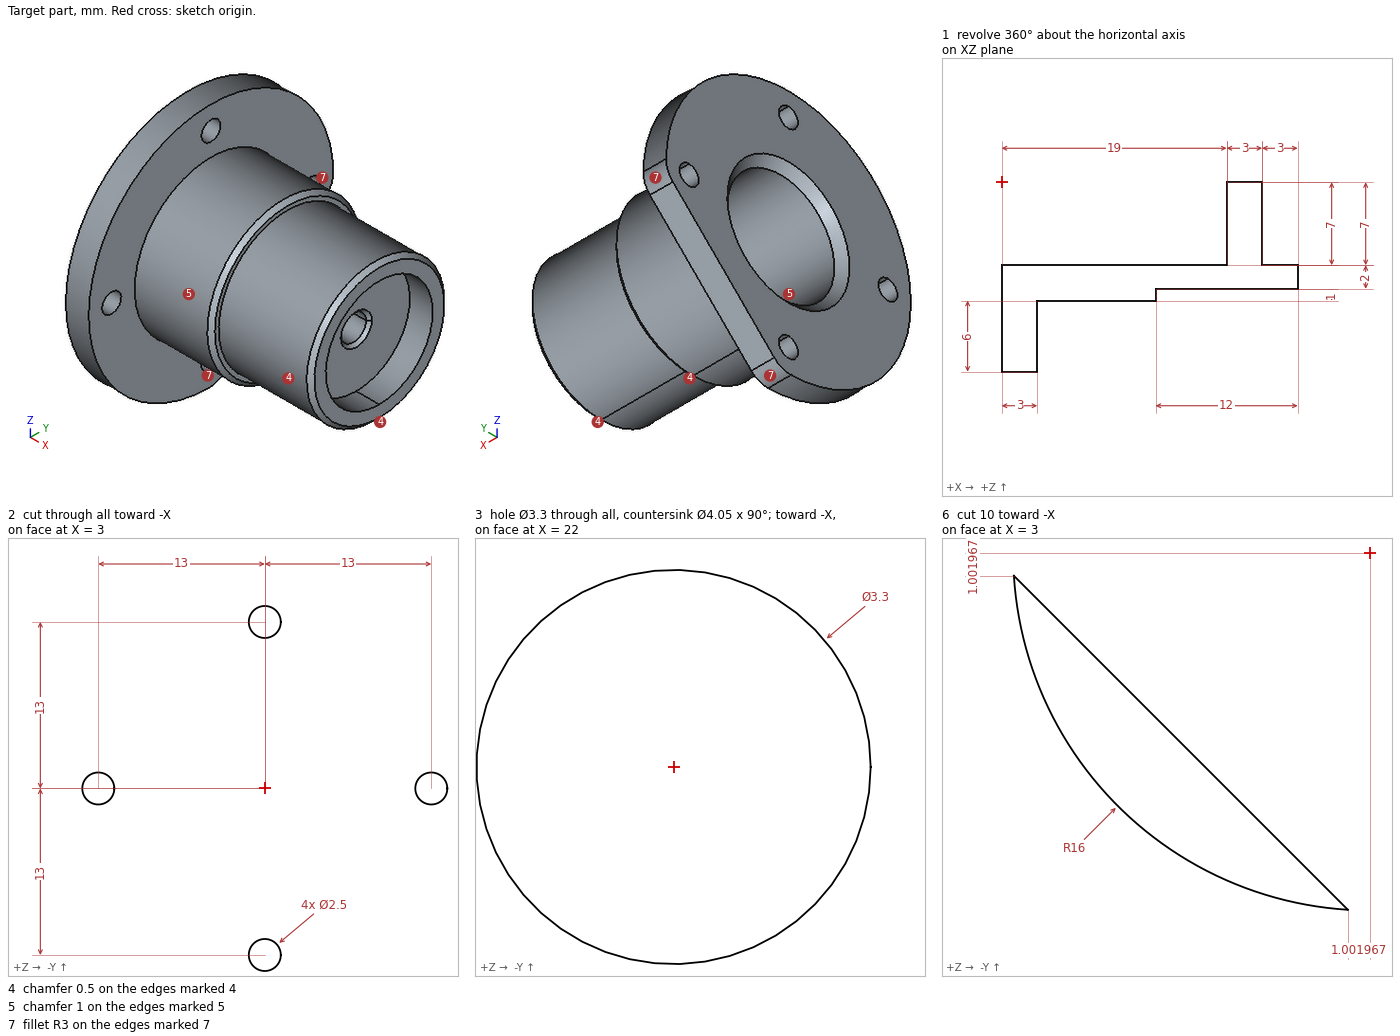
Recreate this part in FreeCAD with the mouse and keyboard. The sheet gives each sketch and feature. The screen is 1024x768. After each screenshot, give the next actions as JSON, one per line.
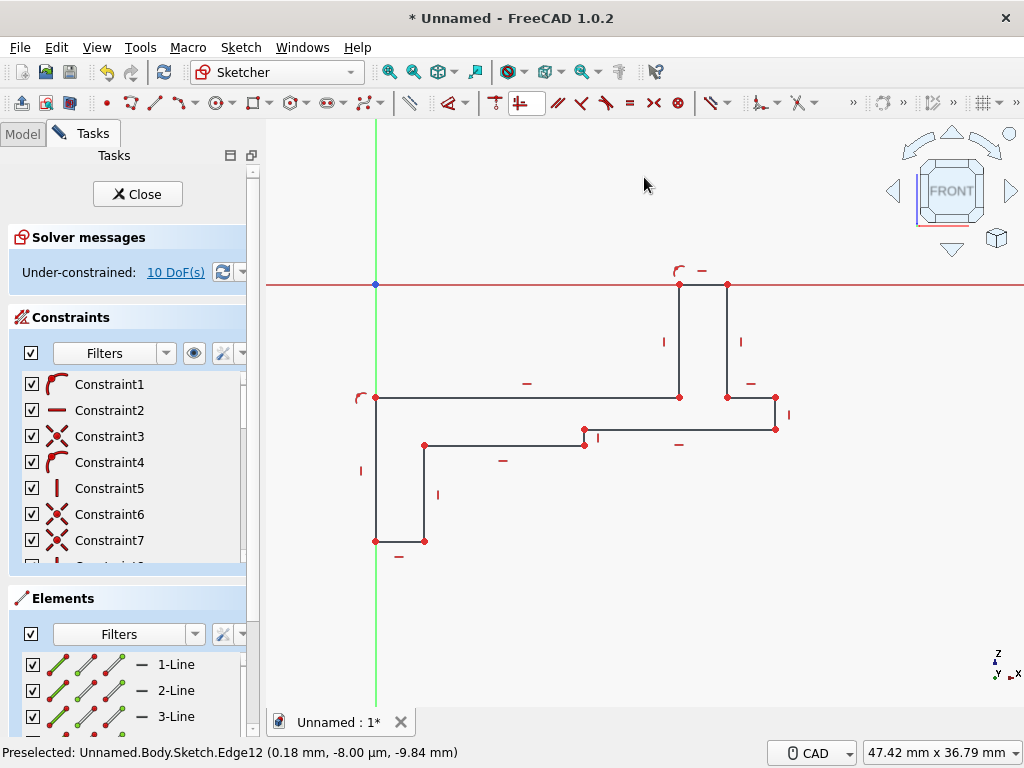
{"action": "left_click", "coordinate": [448, 104]}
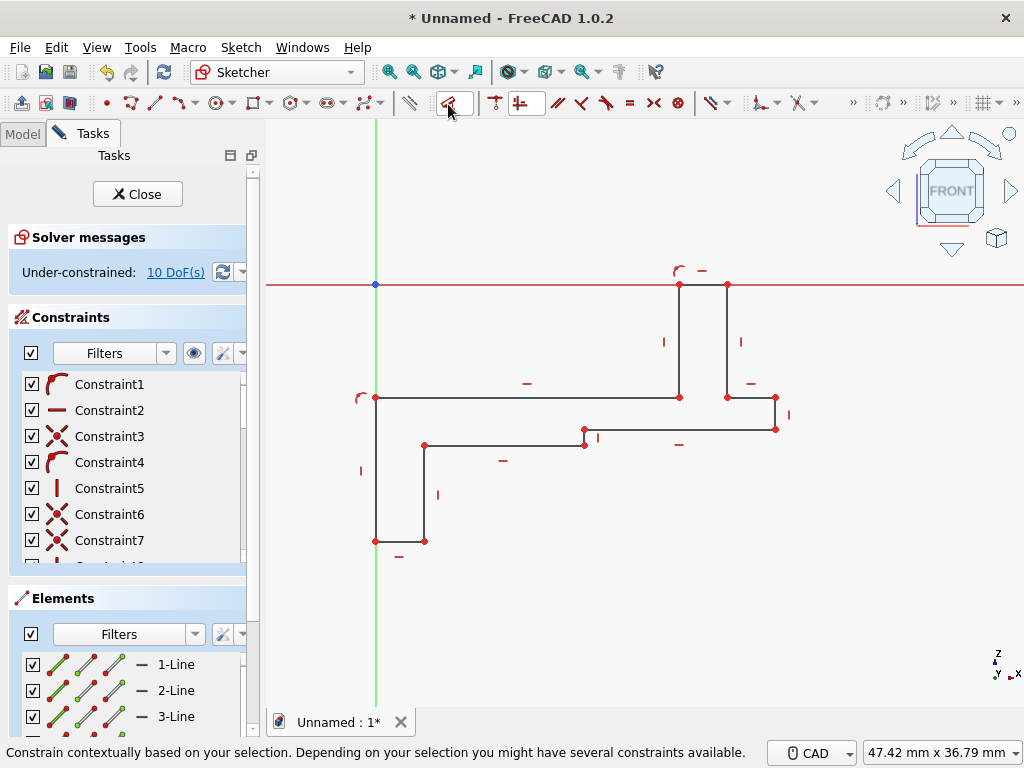
{"action": "left_click", "coordinate": [679, 364]}
{"action": "left_click", "coordinate": [713, 341]}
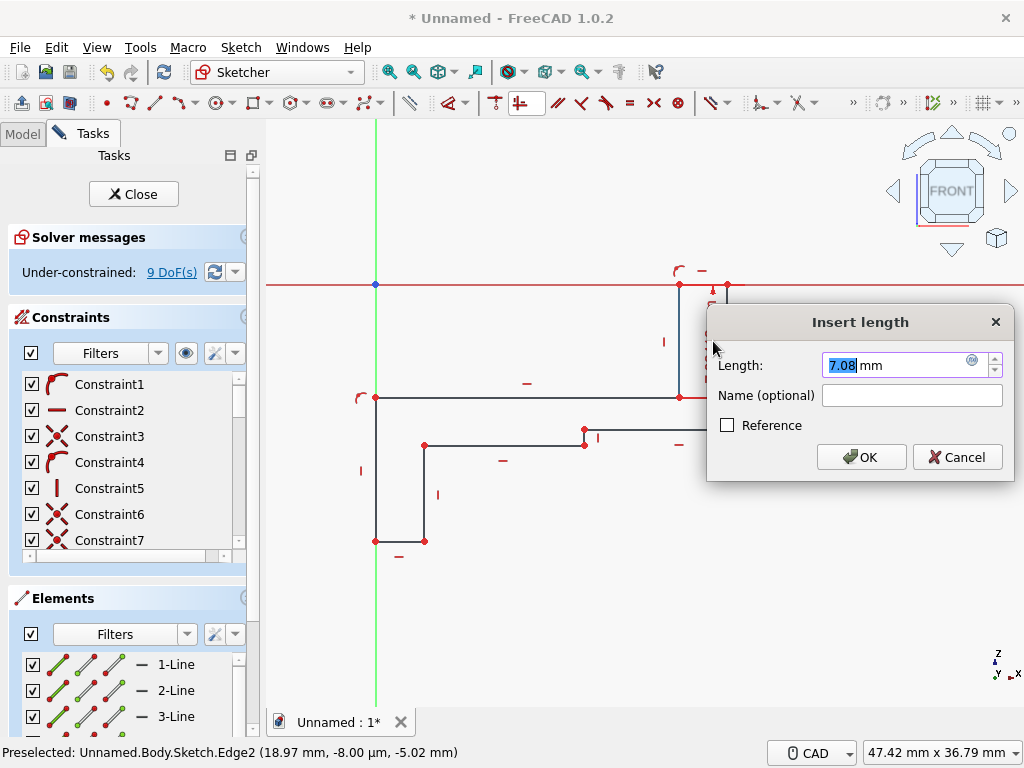
{"action": "type", "text": "7"}
{"action": "key", "text": "Return"}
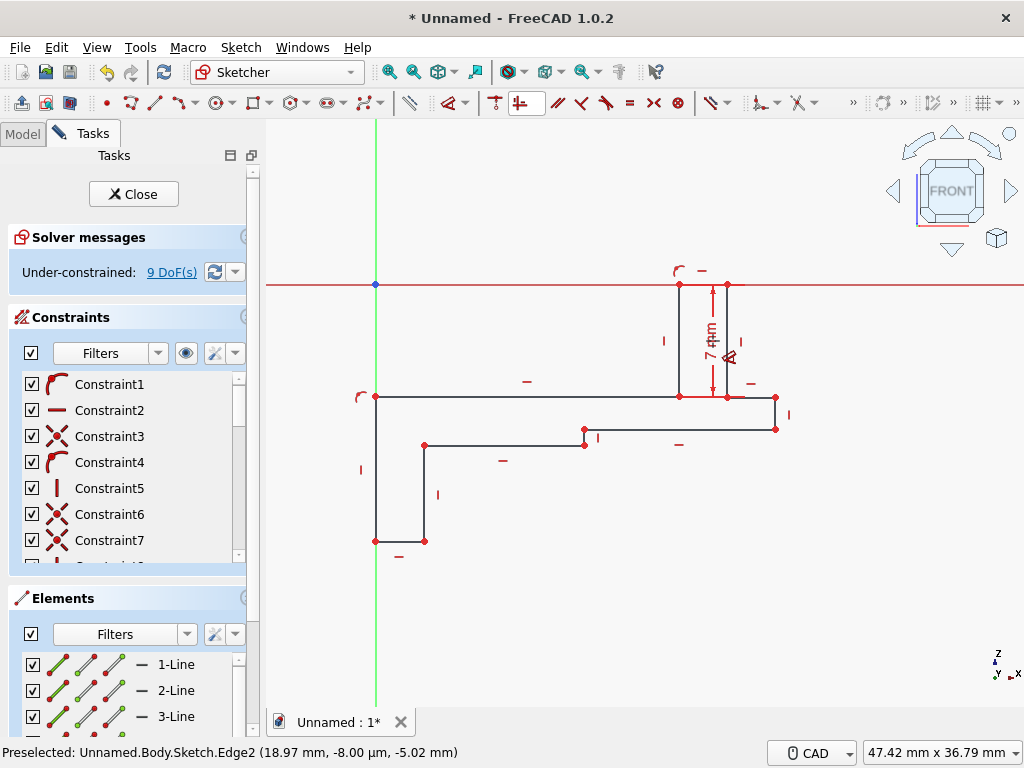
{"action": "left_click", "coordinate": [693, 285]}
{"action": "left_click", "coordinate": [703, 251]}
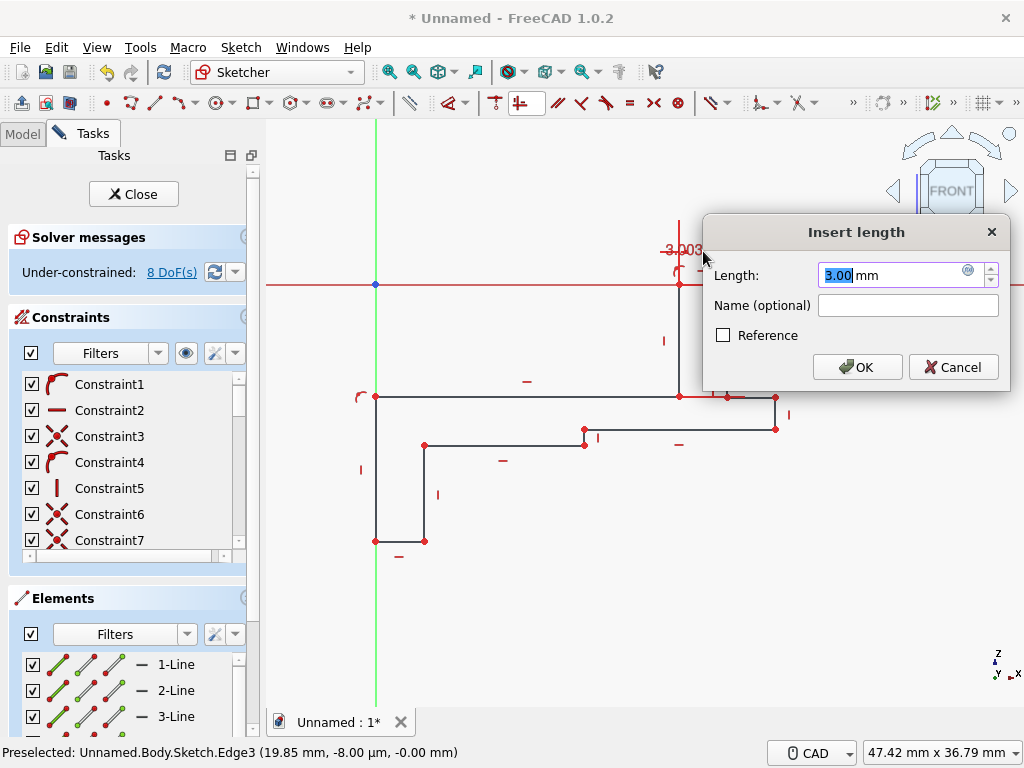
{"action": "type", "text": "3"}
{"action": "key", "text": "Return"}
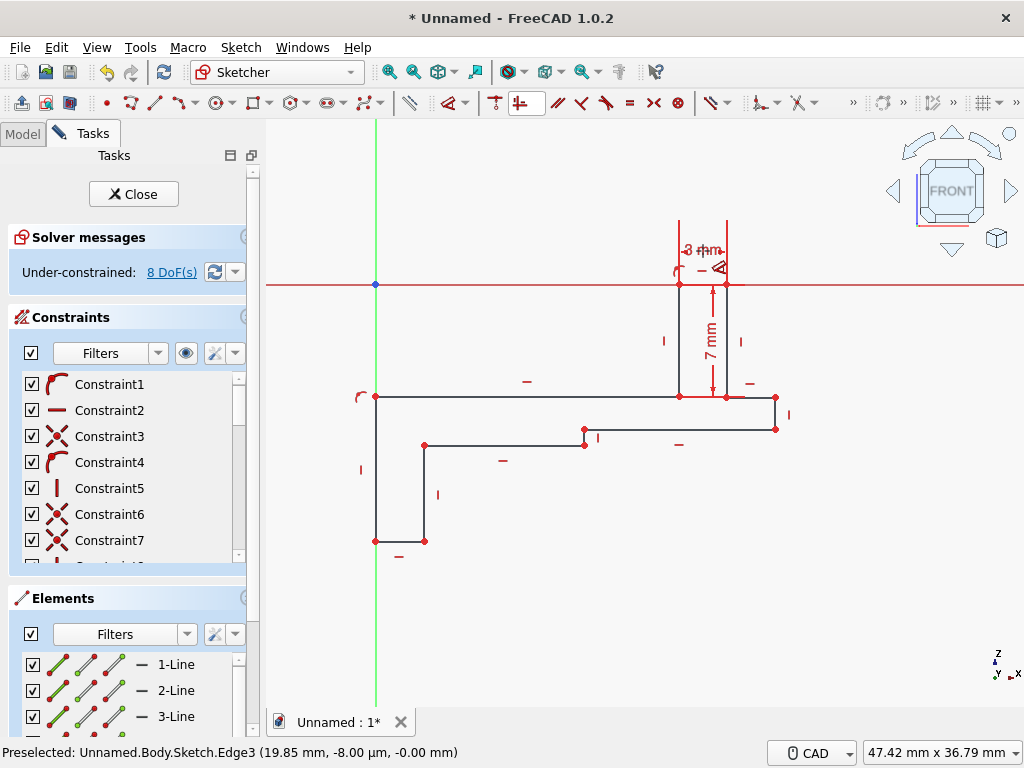
{"action": "left_click", "coordinate": [727, 319]}
{"action": "left_click", "coordinate": [761, 315]}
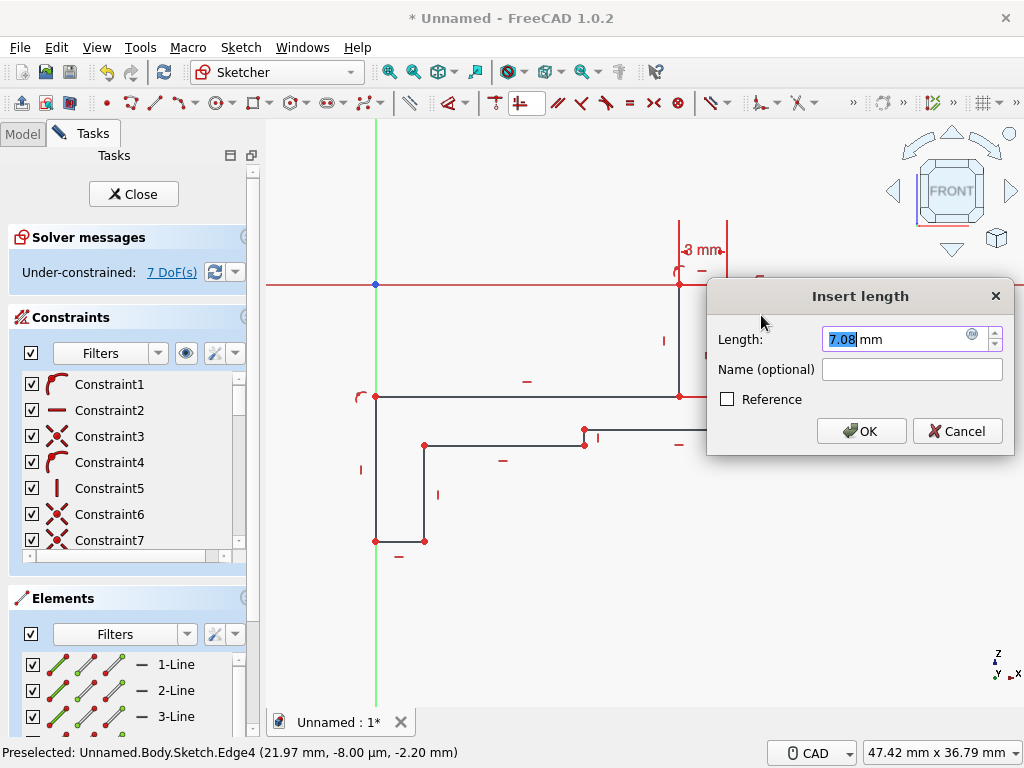
{"action": "type", "text": "7"}
{"action": "key", "text": "Return"}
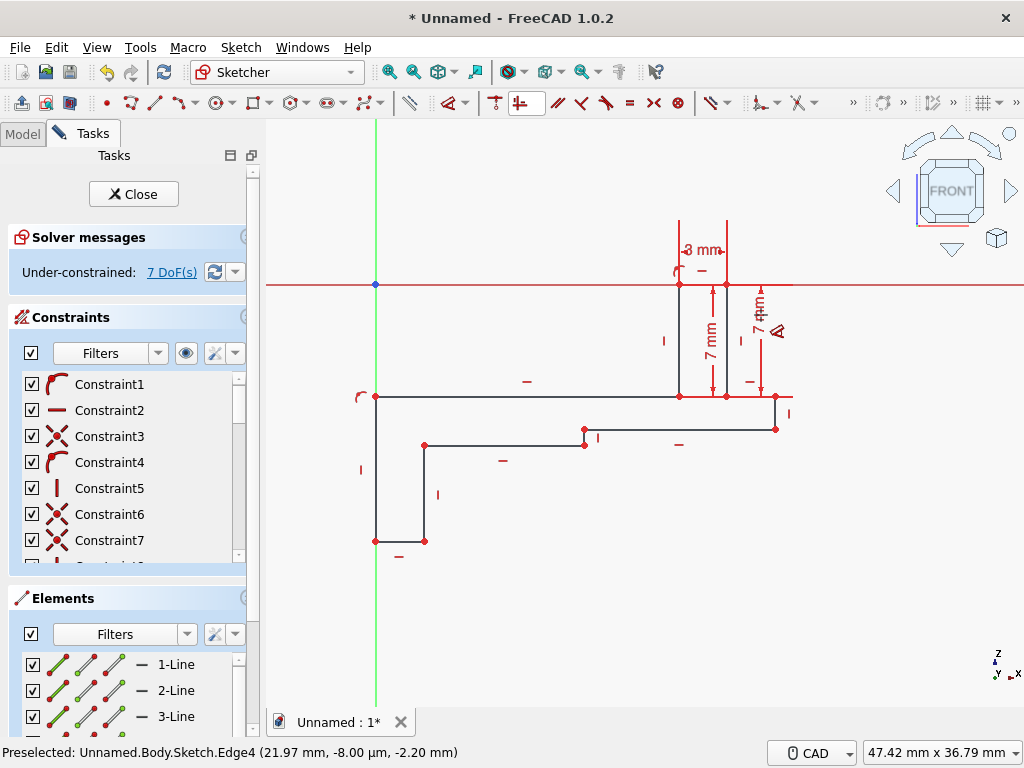
{"action": "left_click", "coordinate": [741, 397]}
{"action": "left_click", "coordinate": [751, 363]}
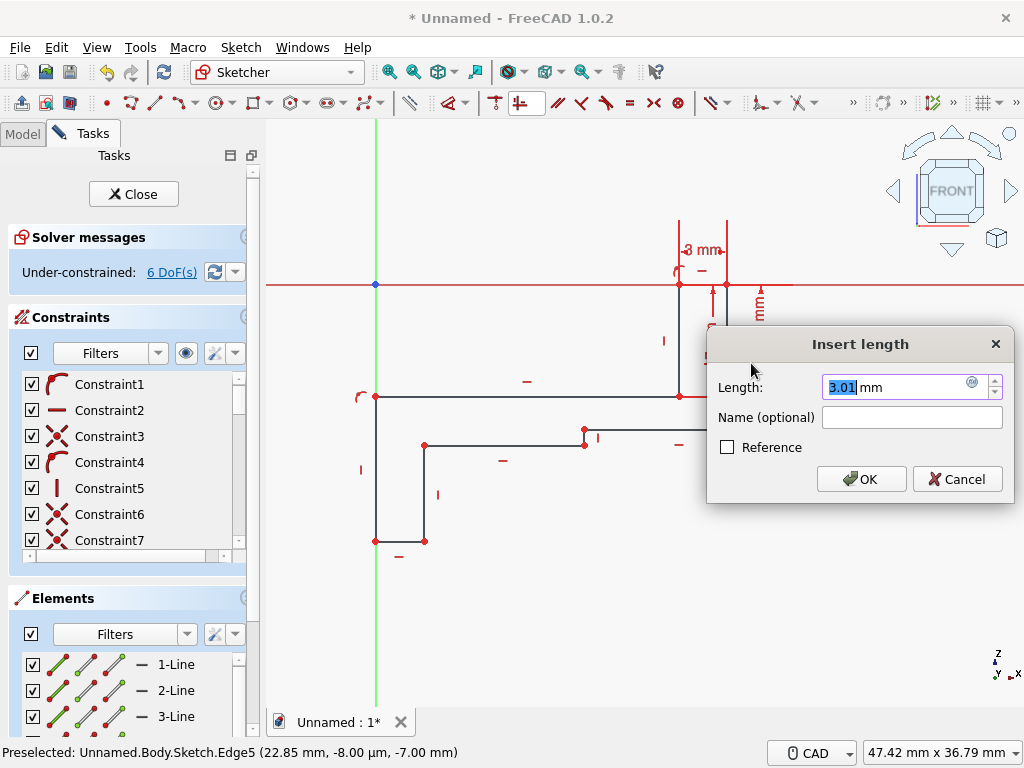
{"action": "type", "text": "3"}
{"action": "key", "text": "Return"}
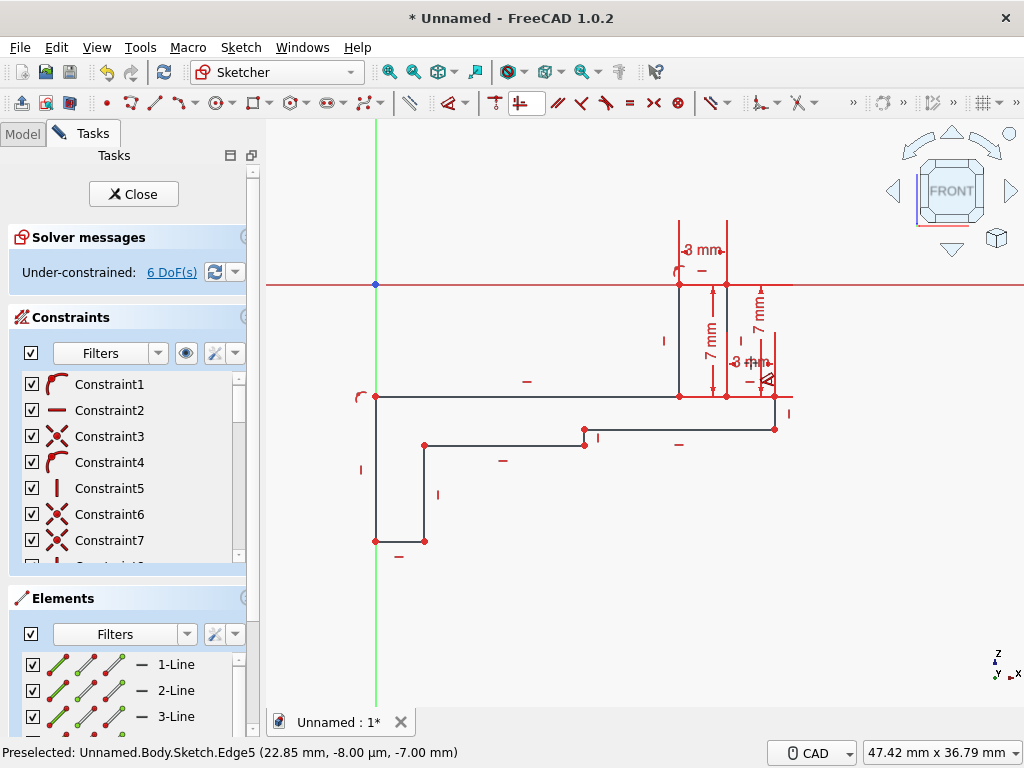
{"action": "scroll", "coordinate": [775, 407], "scroll_direction": "up", "scroll_amount": 2}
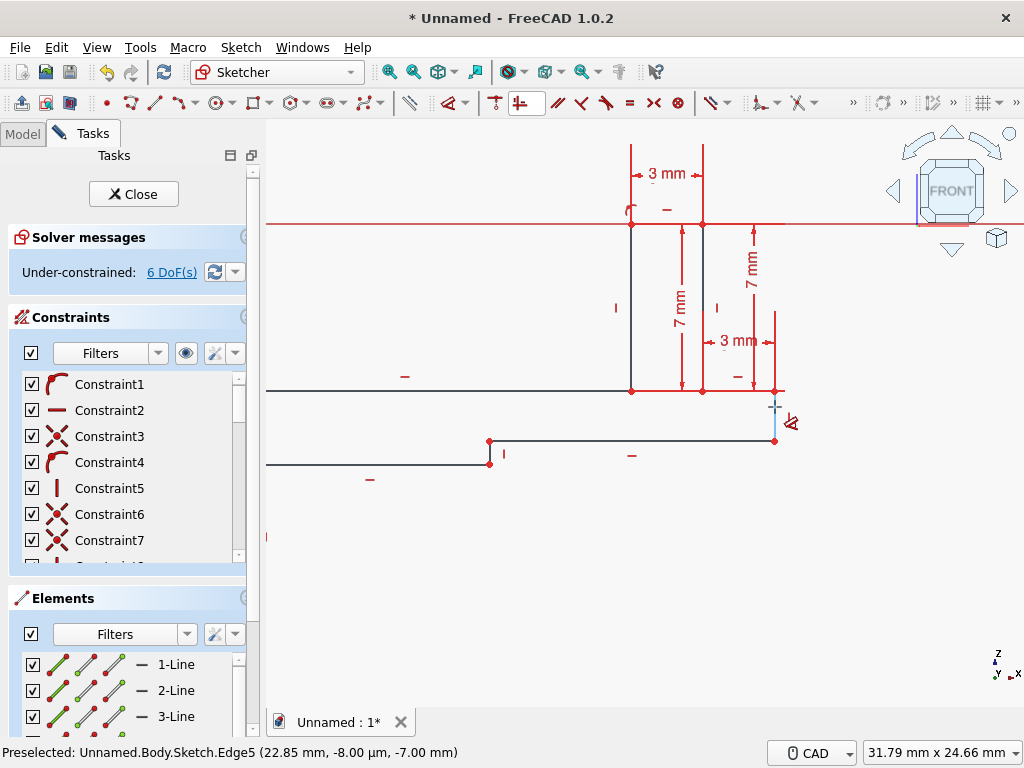
{"action": "left_click", "coordinate": [775, 406]}
{"action": "left_click", "coordinate": [809, 416]}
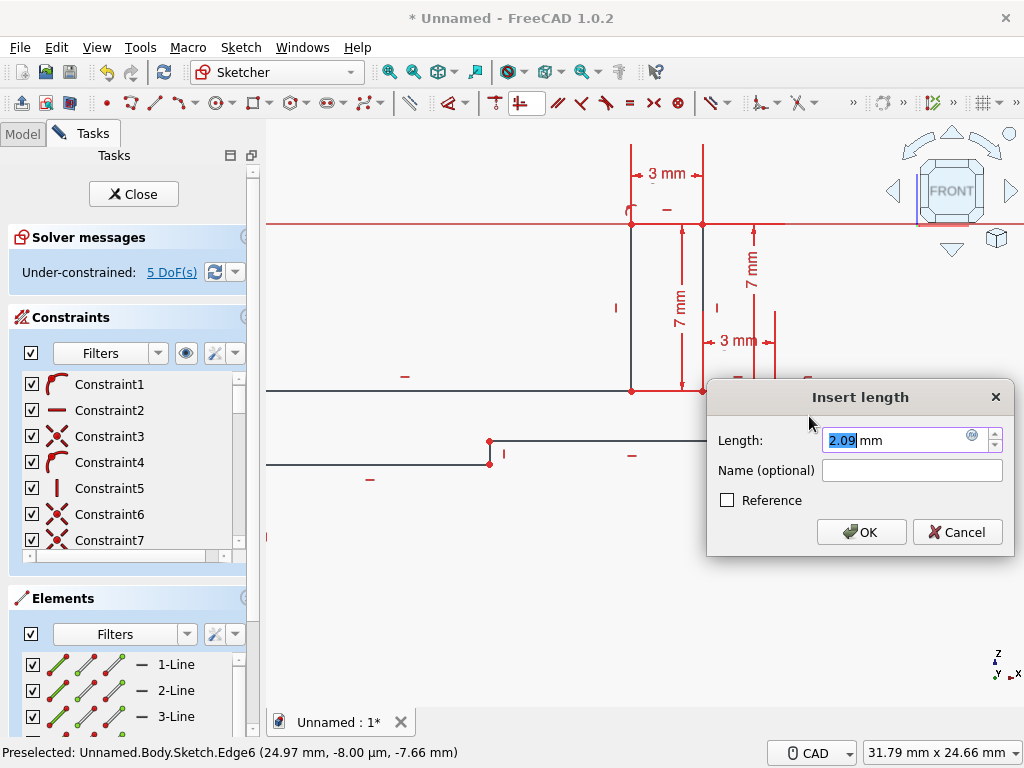
{"action": "type", "text": "2"}
{"action": "key", "text": "Return"}